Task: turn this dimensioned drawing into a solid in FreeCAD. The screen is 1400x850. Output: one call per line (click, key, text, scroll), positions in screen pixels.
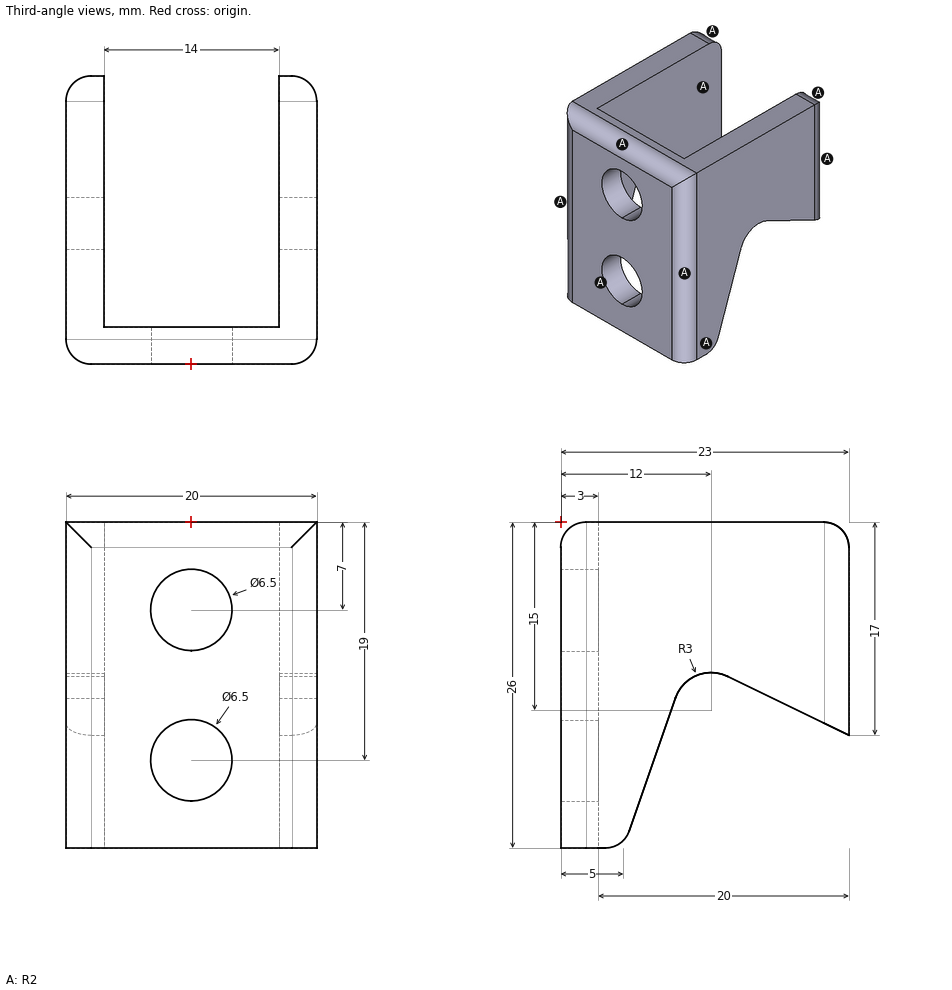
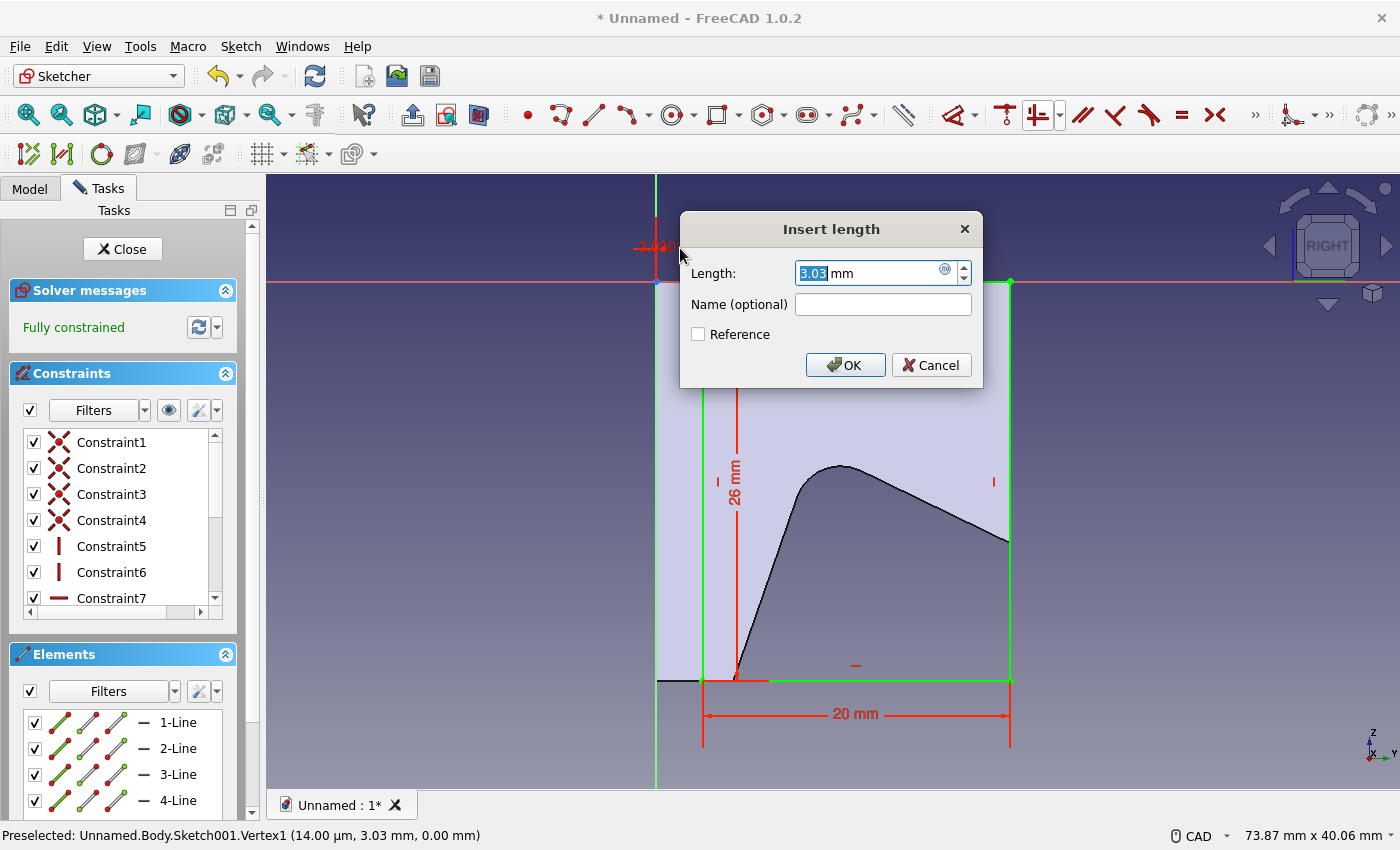
text(3)
key(Return)
key(Escape)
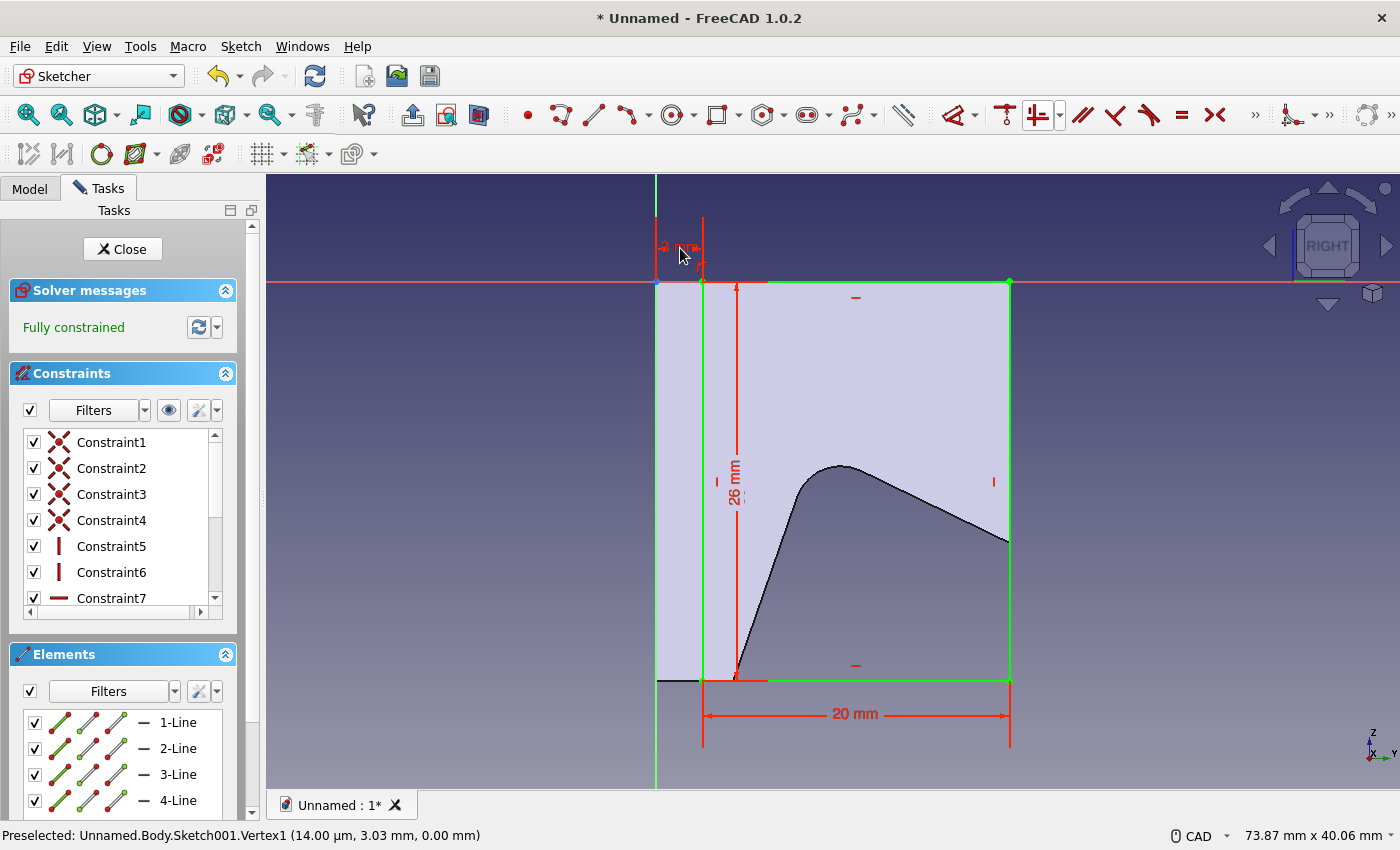
click(123, 249)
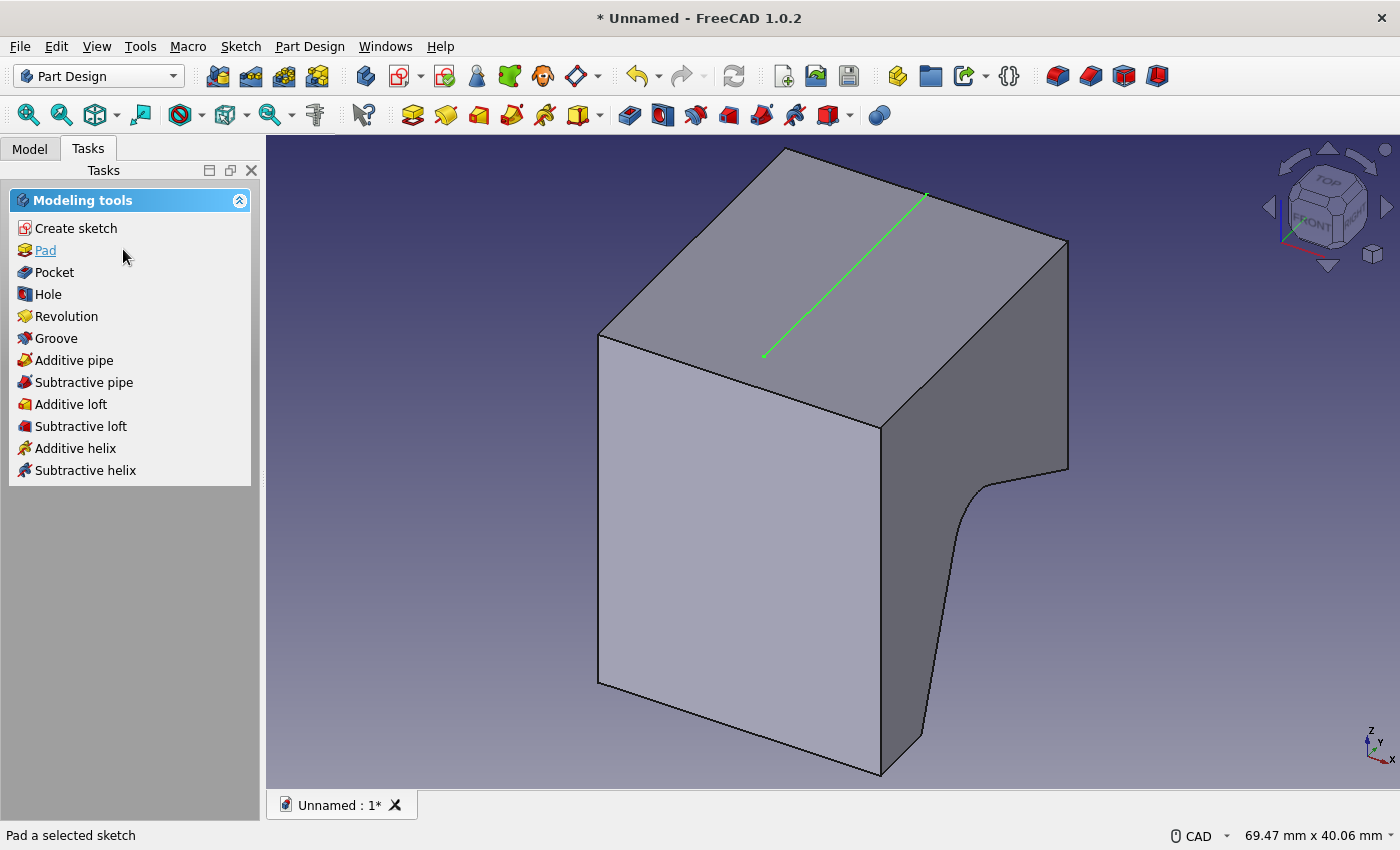
click(630, 116)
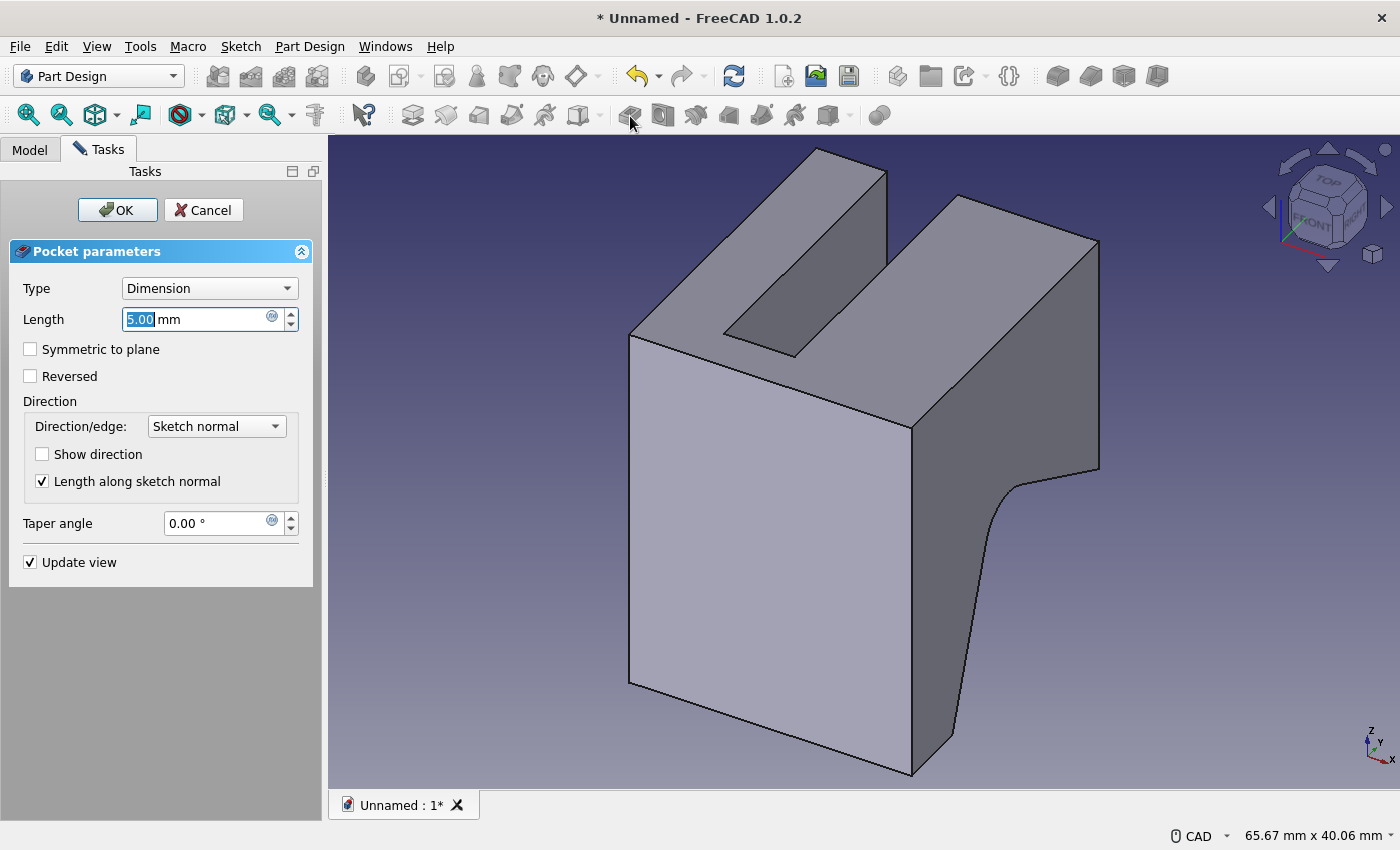
text(14)
key(Tab)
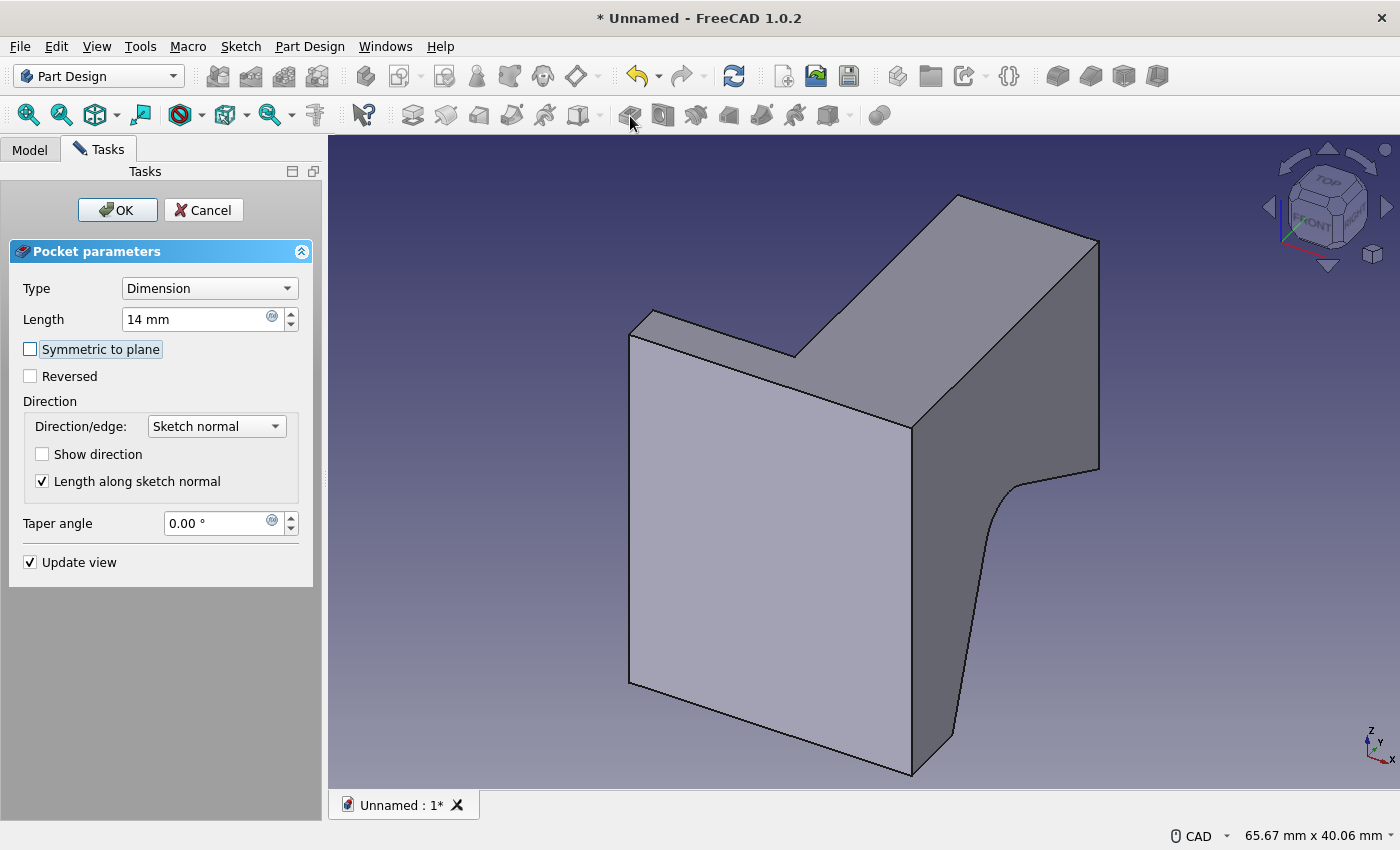
click(31, 349)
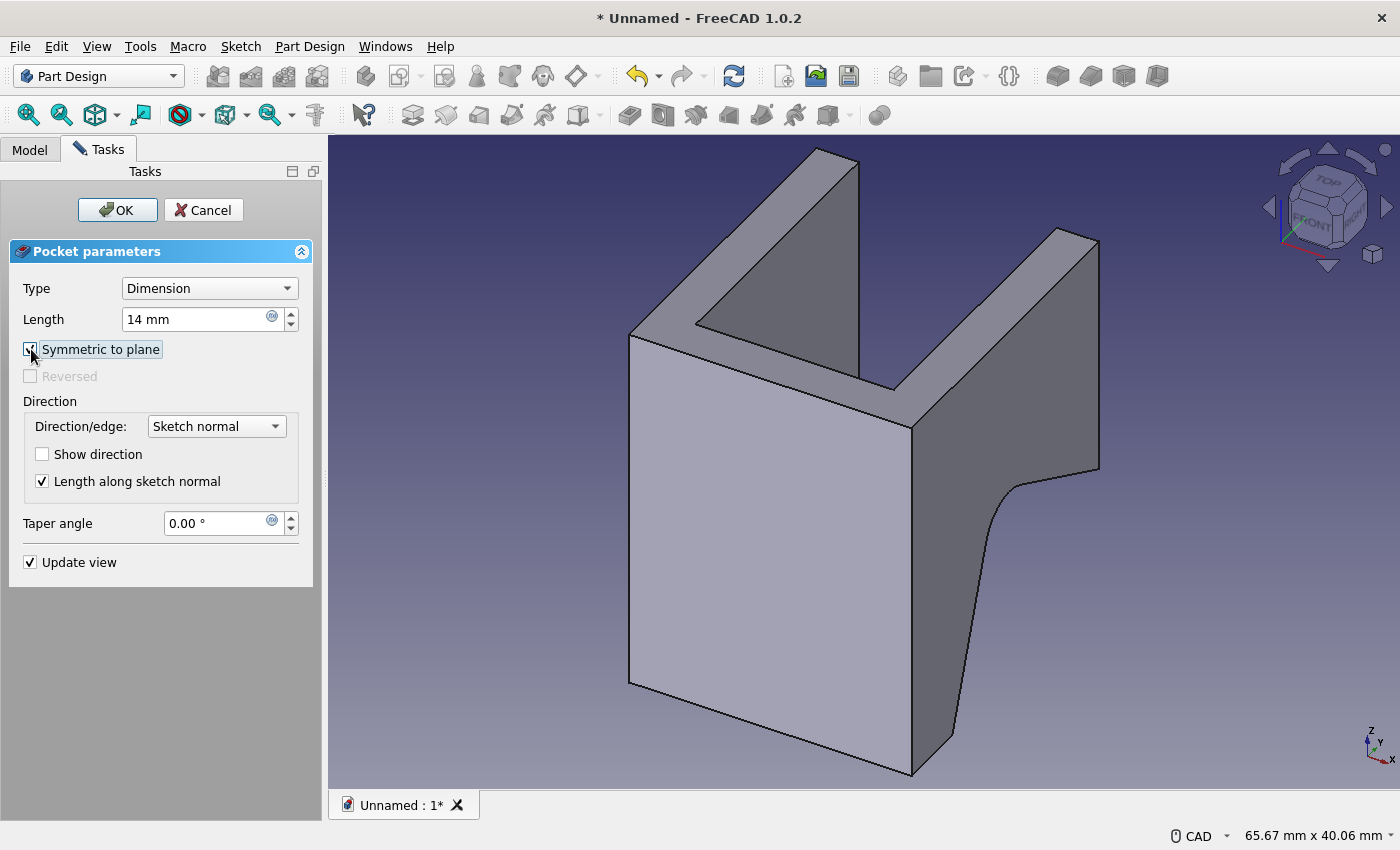
click(118, 210)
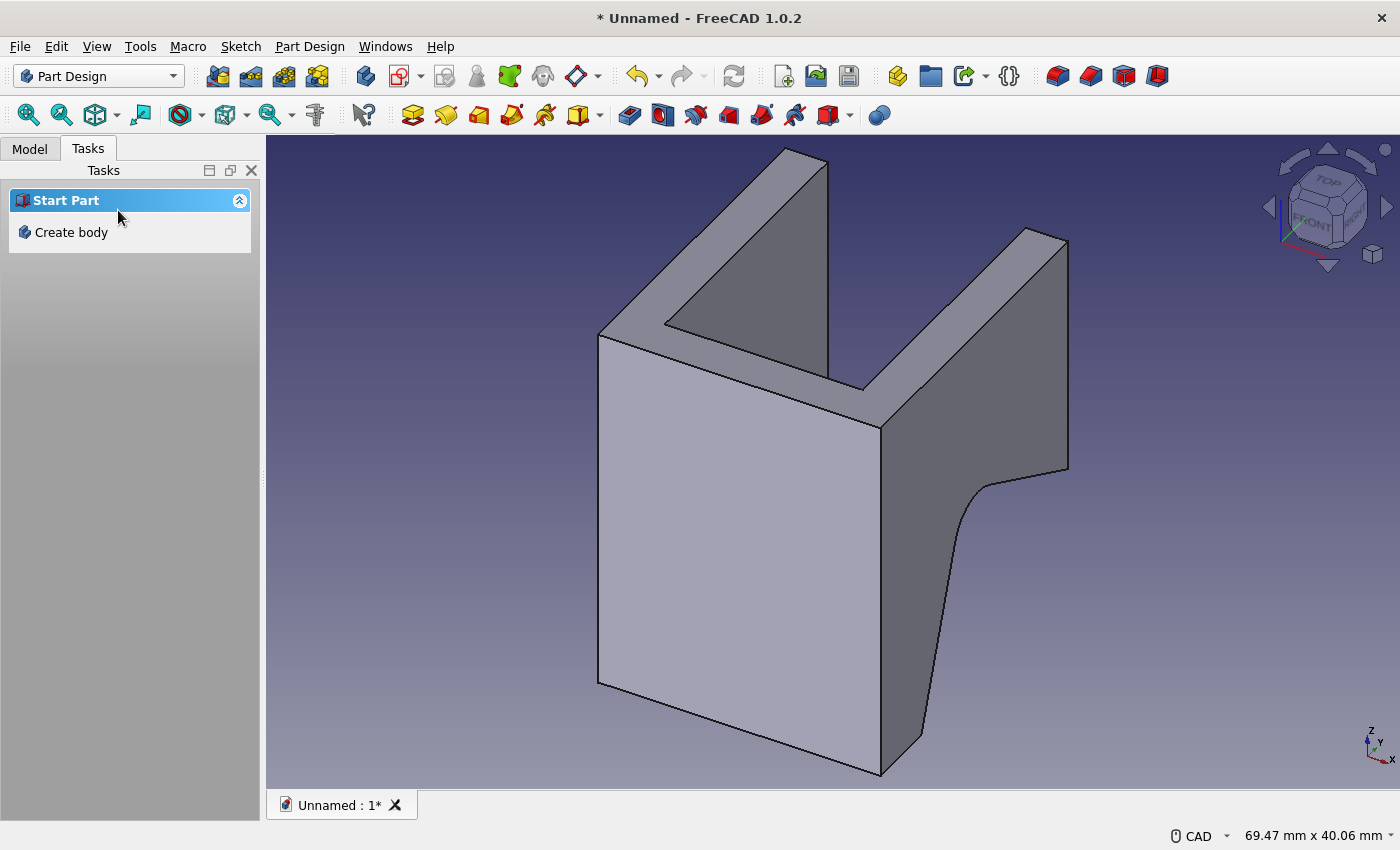
click(739, 554)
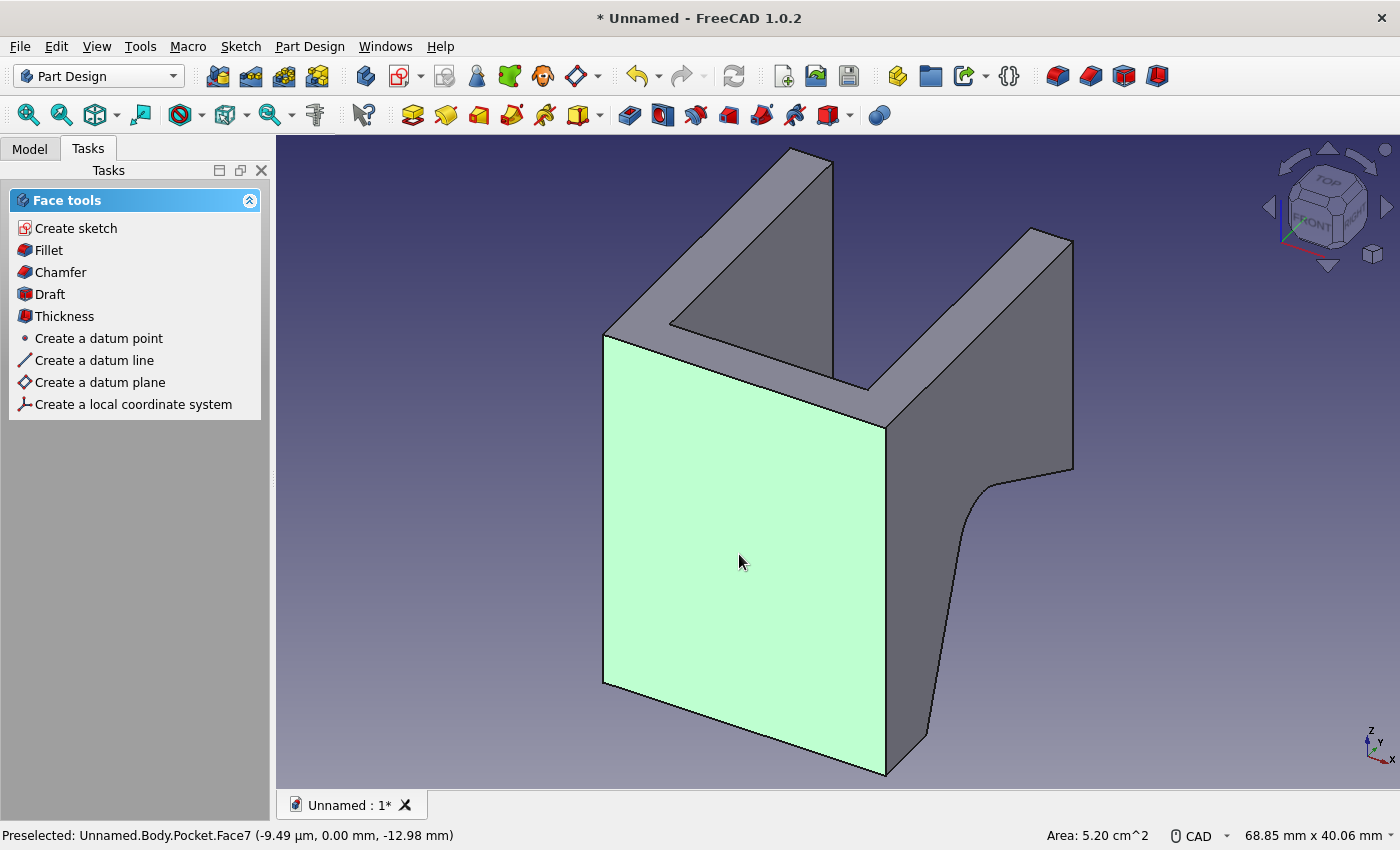
click(398, 76)